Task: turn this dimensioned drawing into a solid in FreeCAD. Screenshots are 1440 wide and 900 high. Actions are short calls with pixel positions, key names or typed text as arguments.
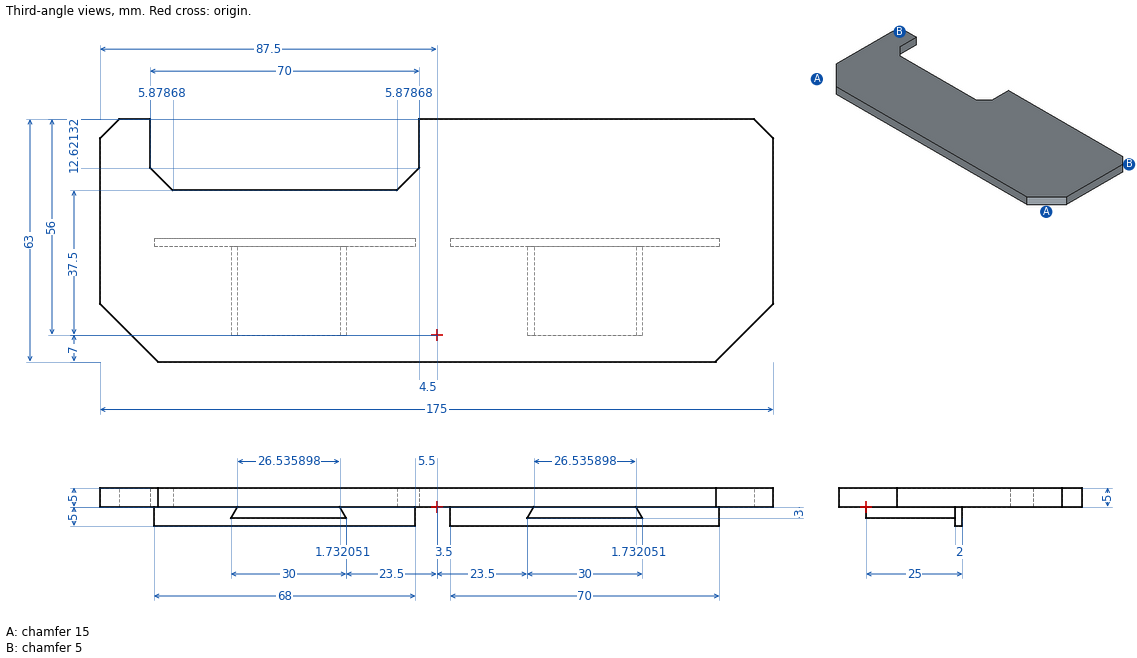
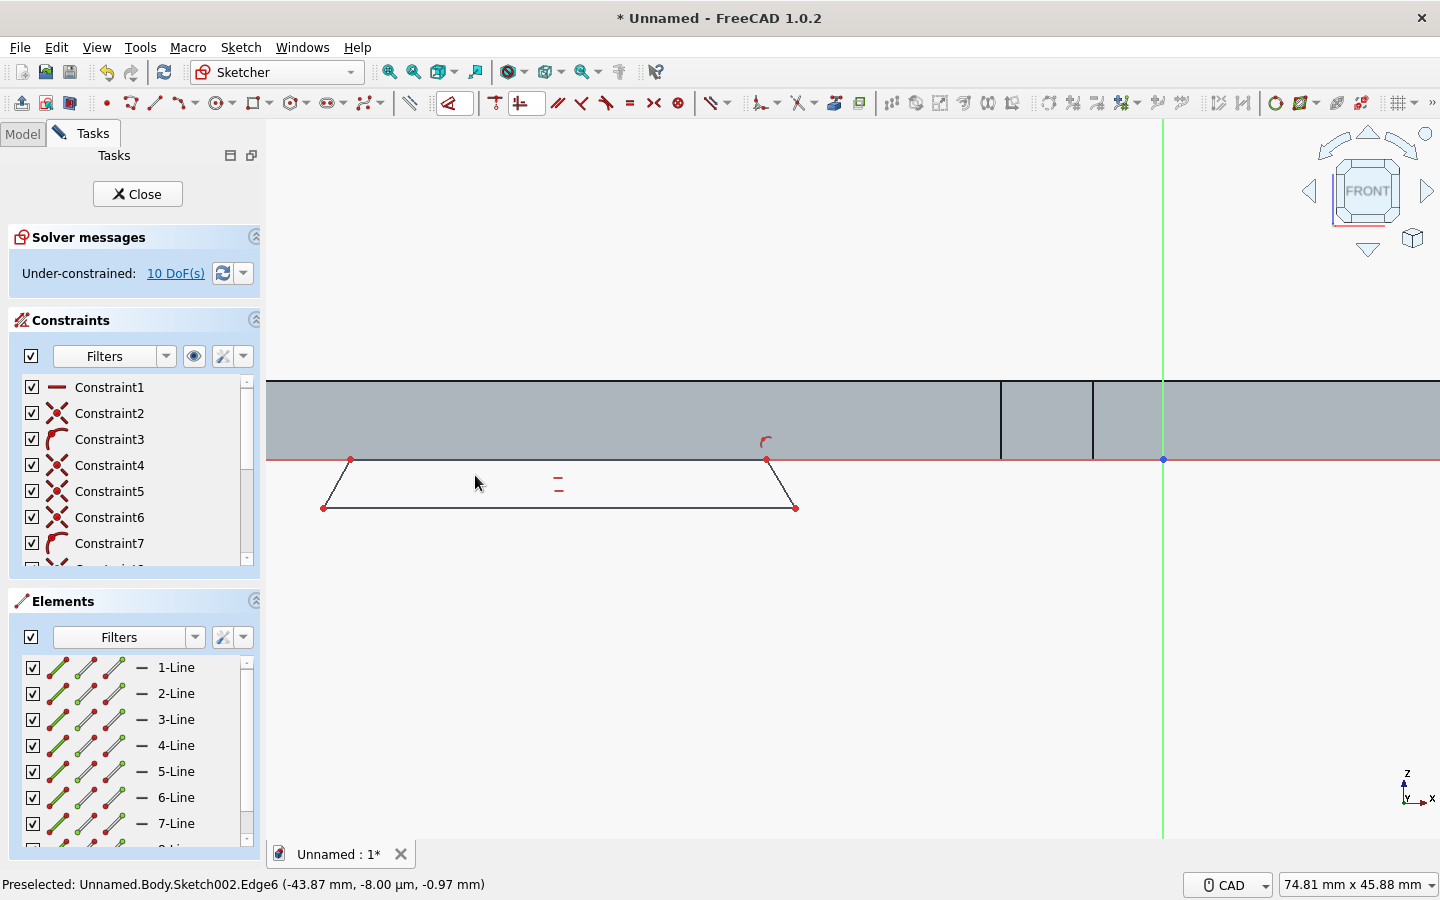
scroll(475, 475, down, 4)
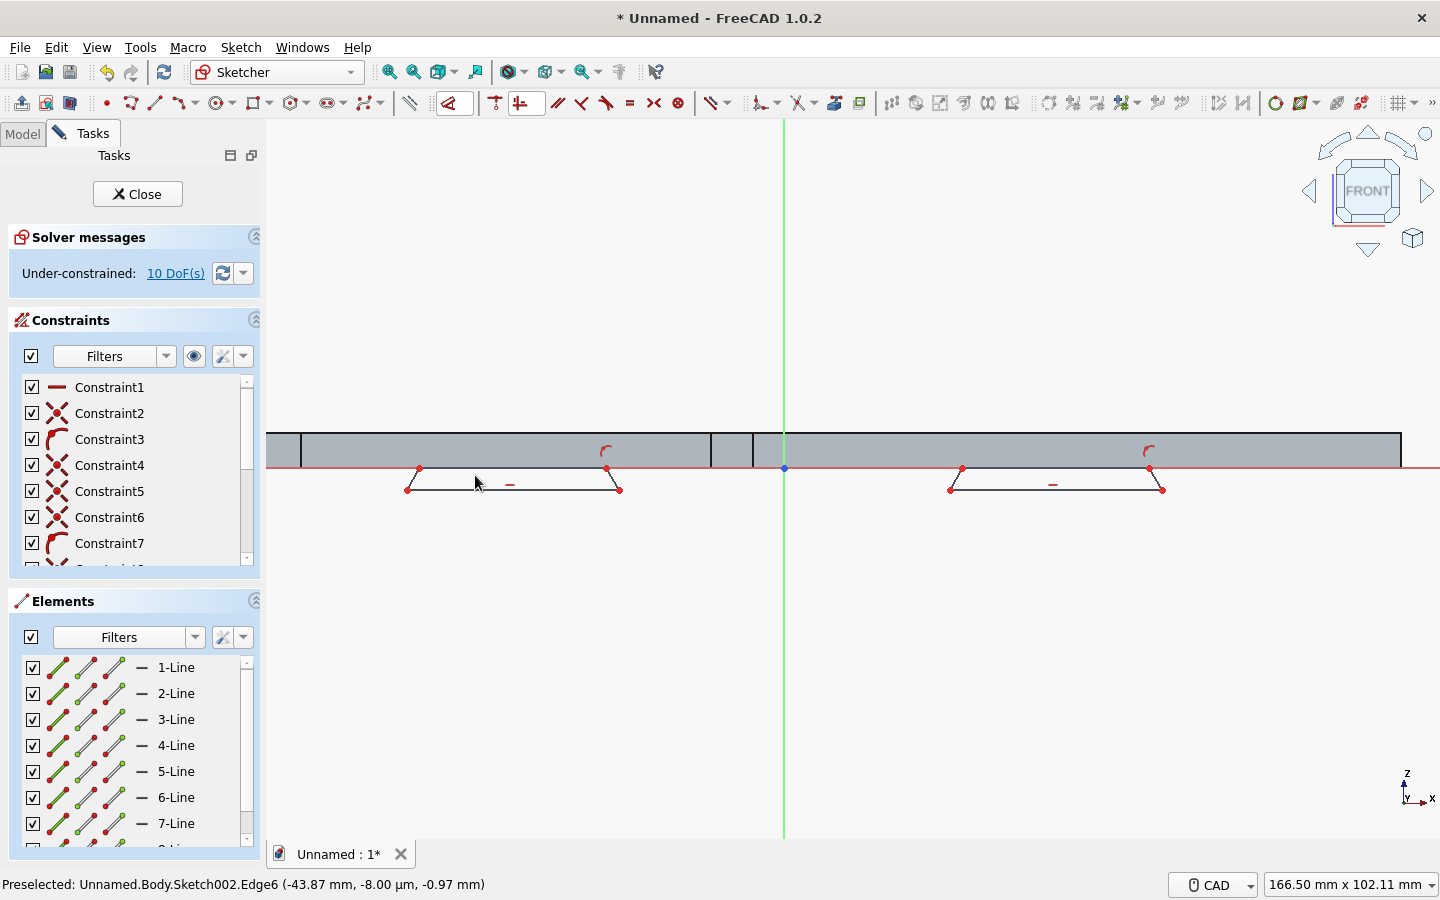
click(1014, 490)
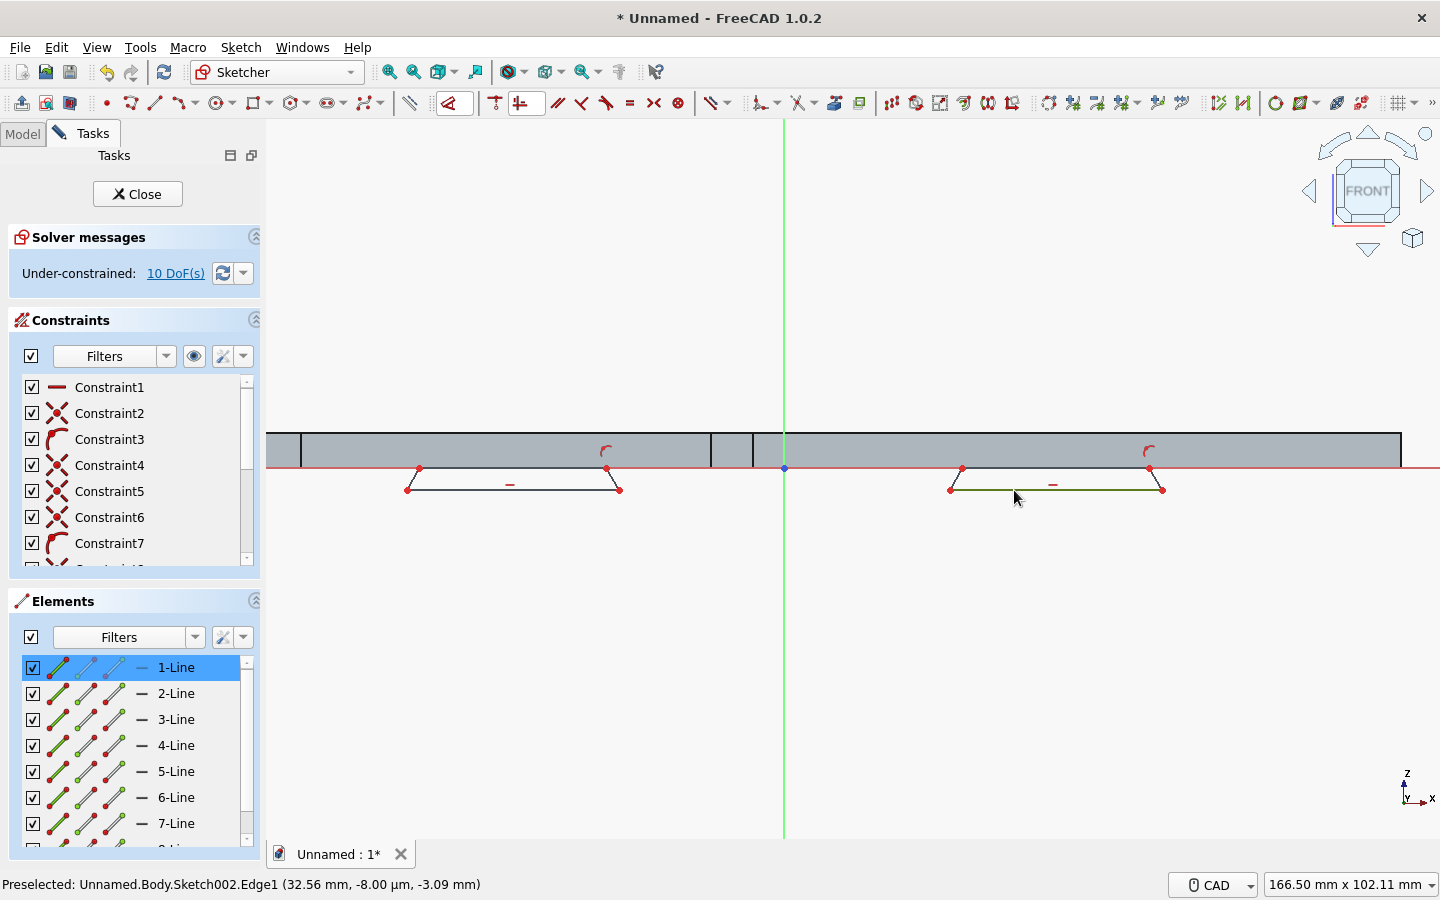
click(468, 104)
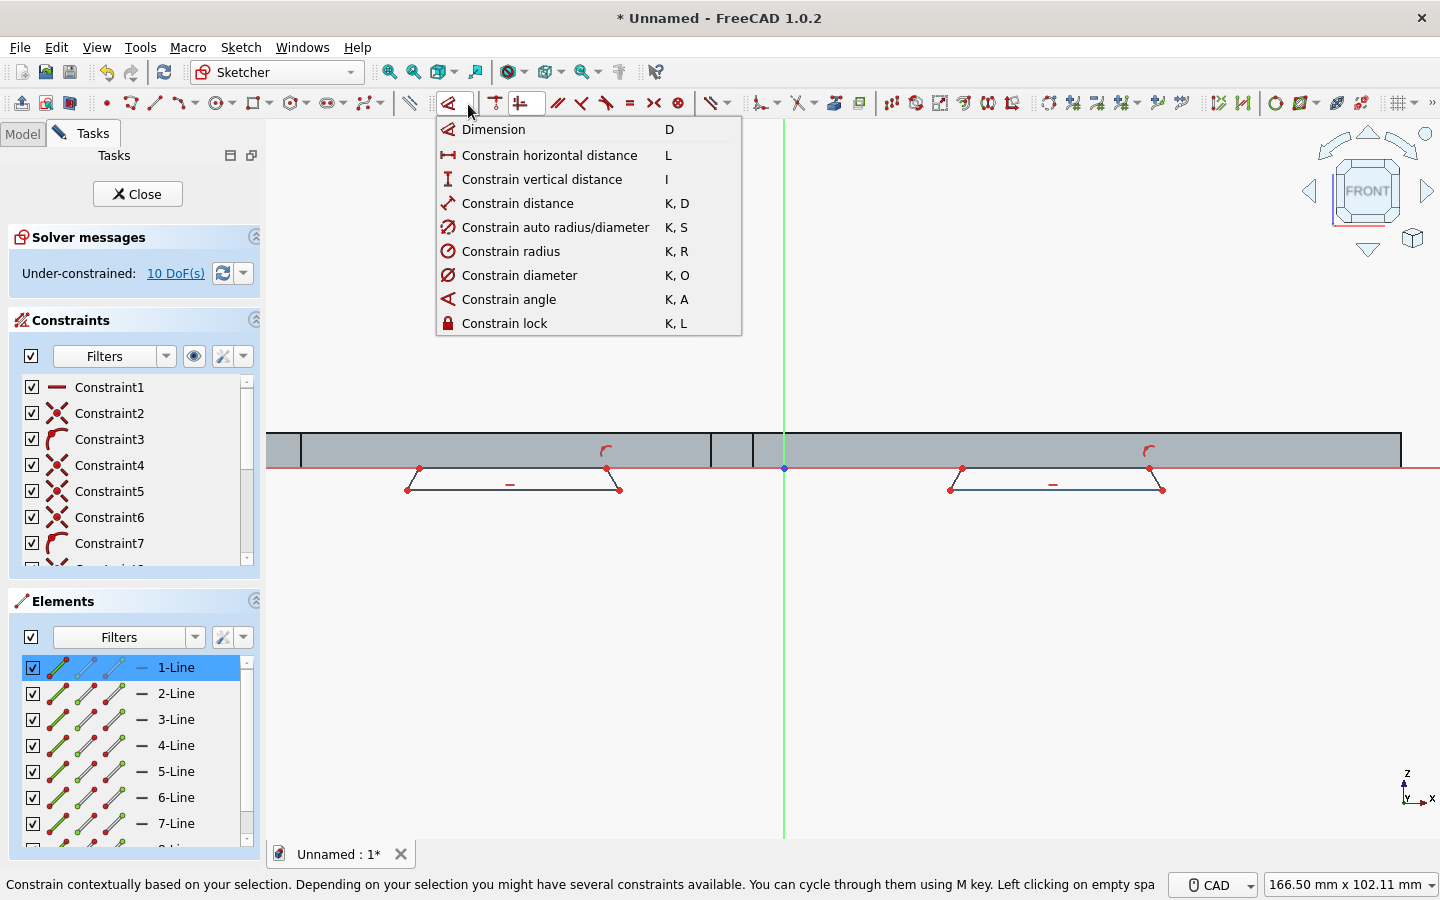
click(589, 155)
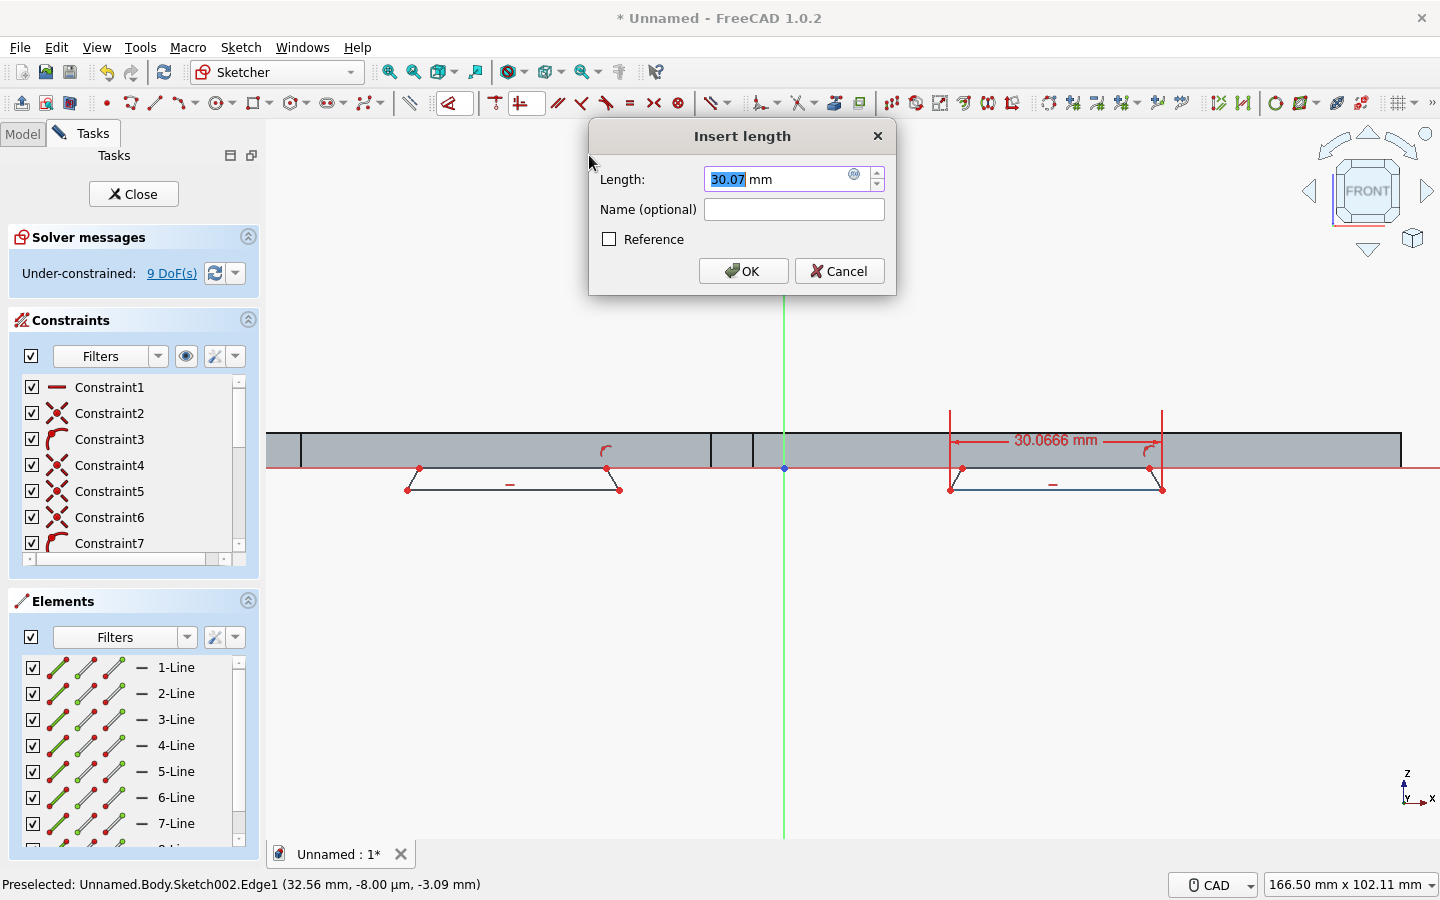
text(30)
key(Return)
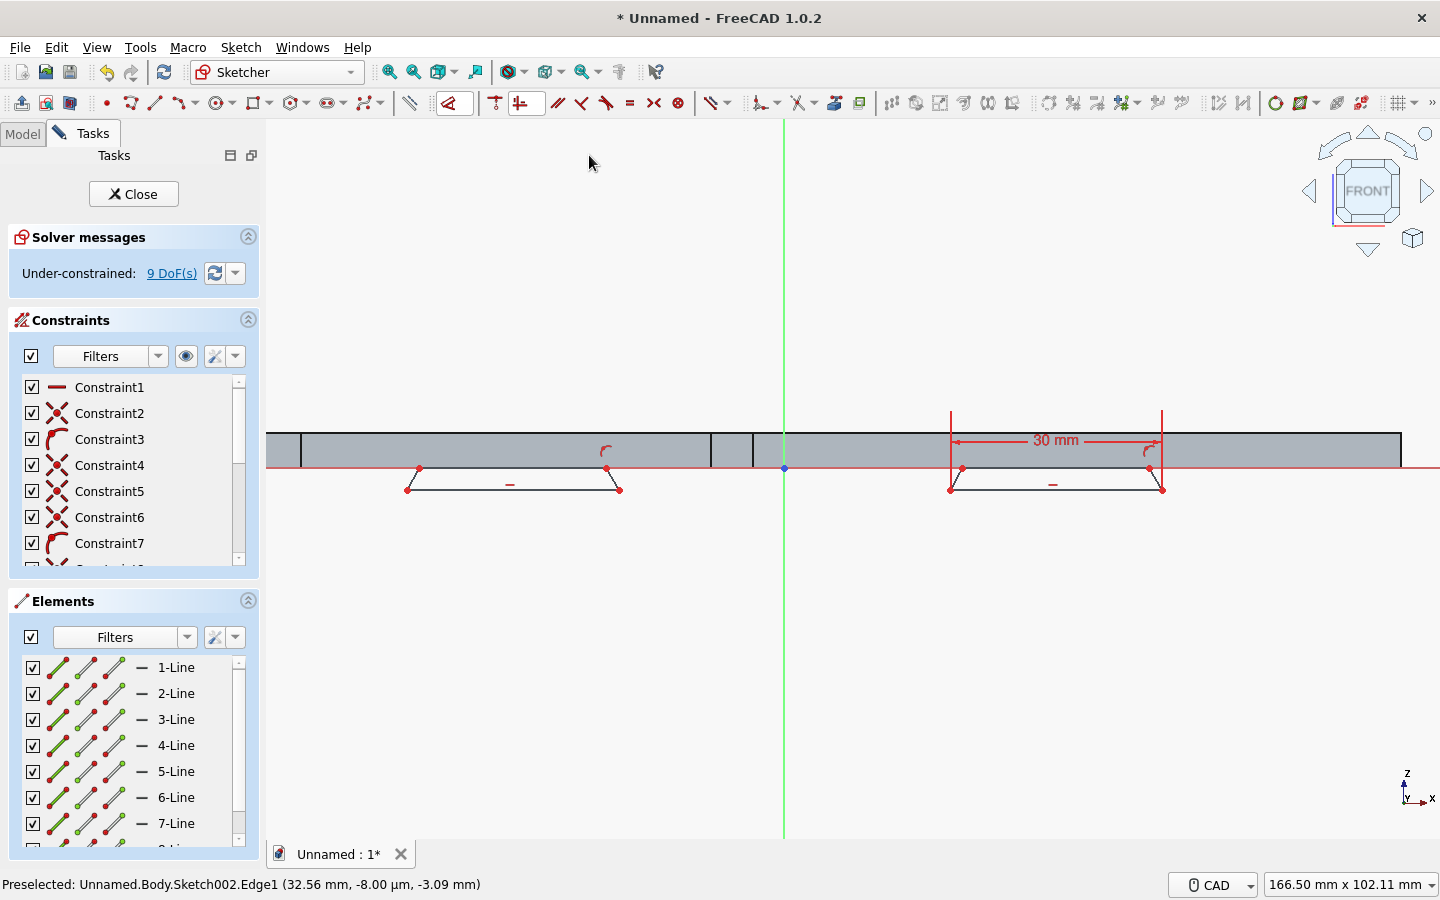
click(471, 490)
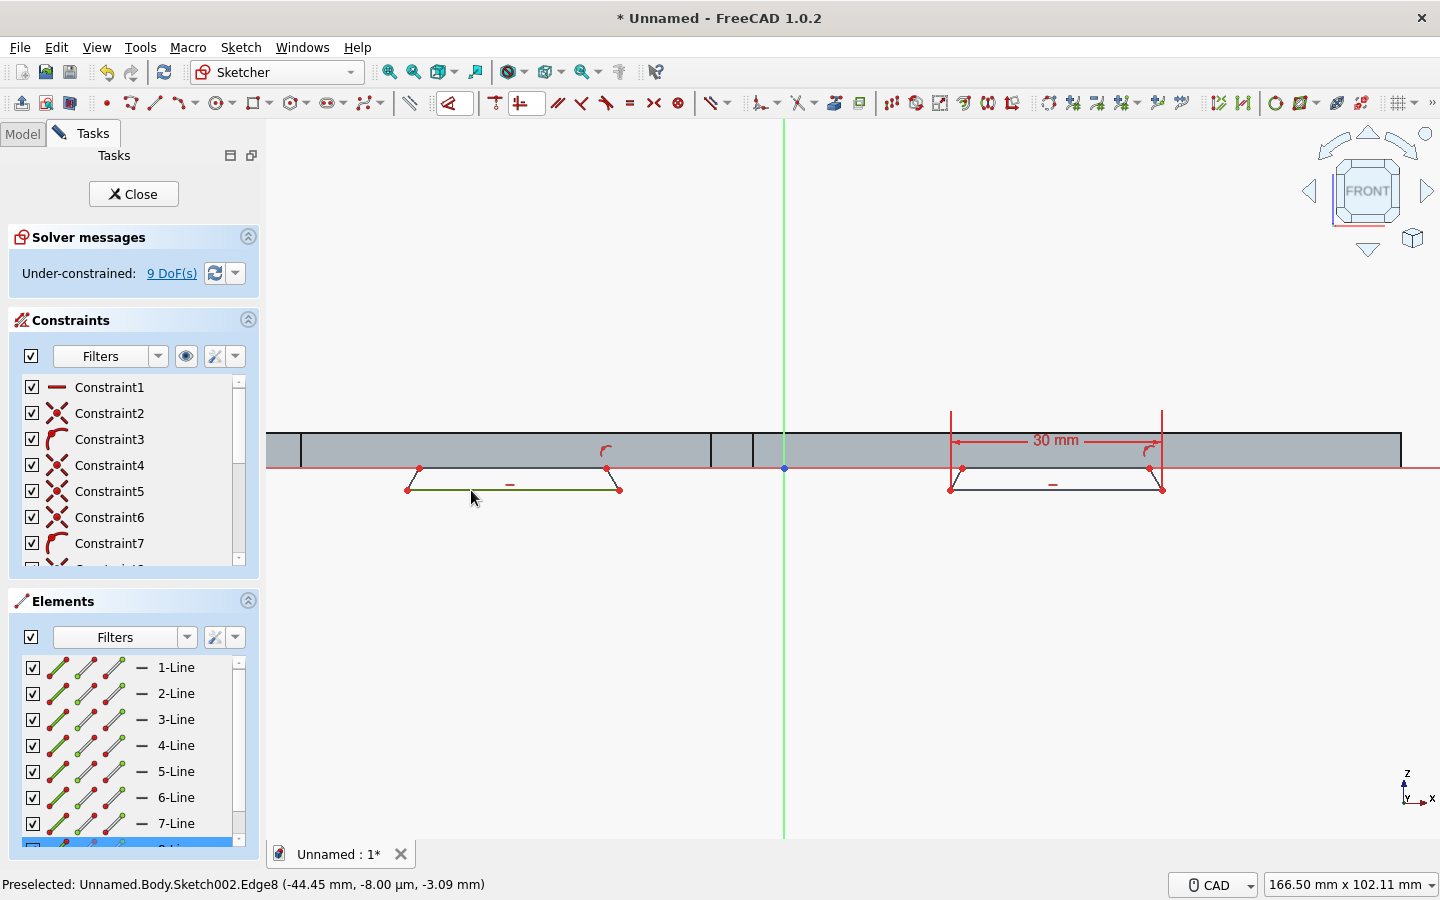
click(468, 104)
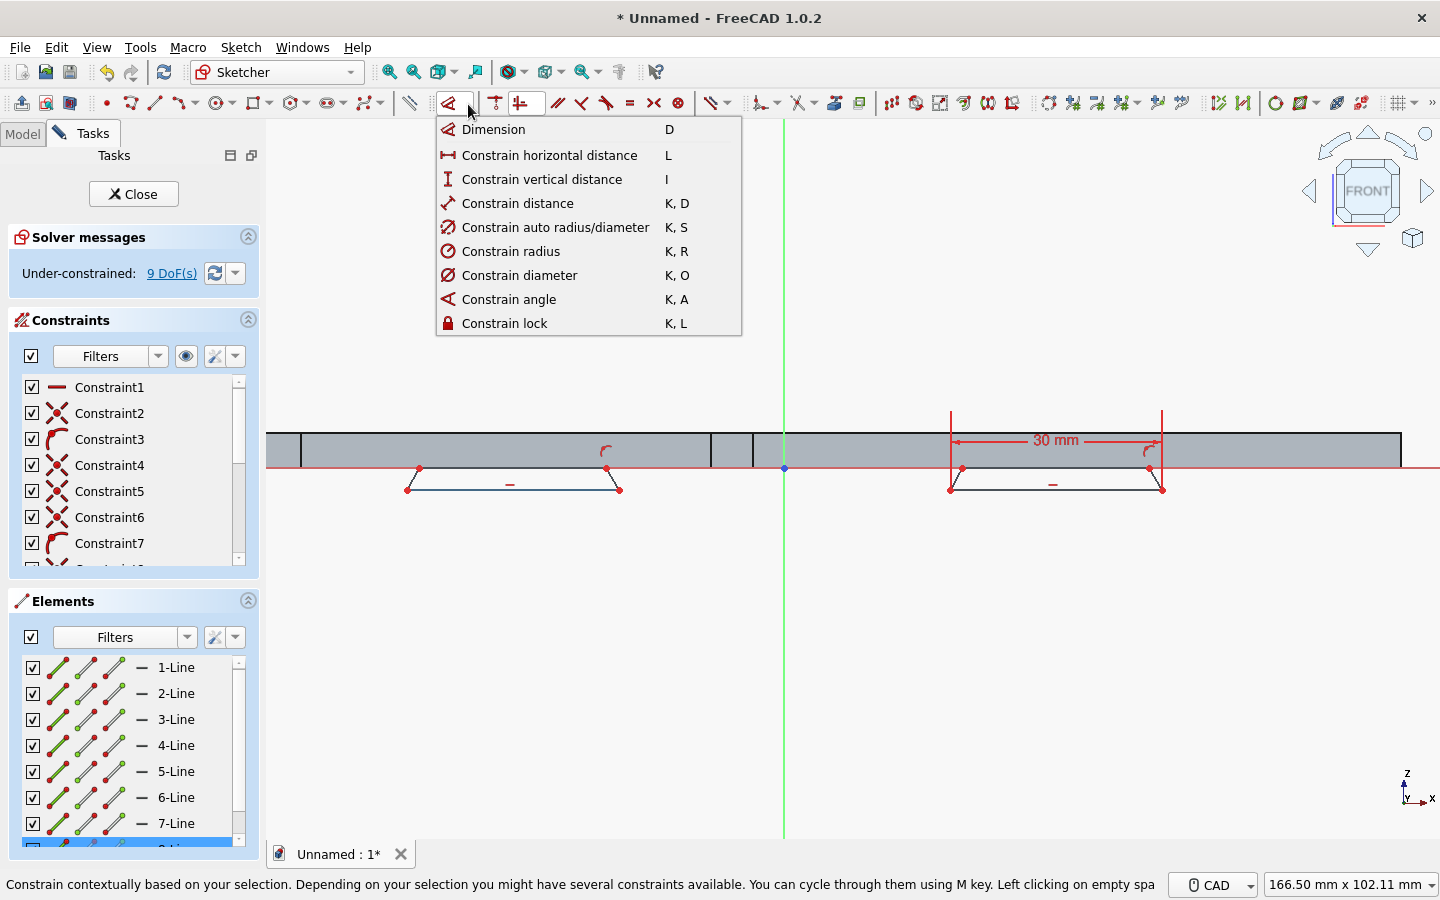
click(589, 155)